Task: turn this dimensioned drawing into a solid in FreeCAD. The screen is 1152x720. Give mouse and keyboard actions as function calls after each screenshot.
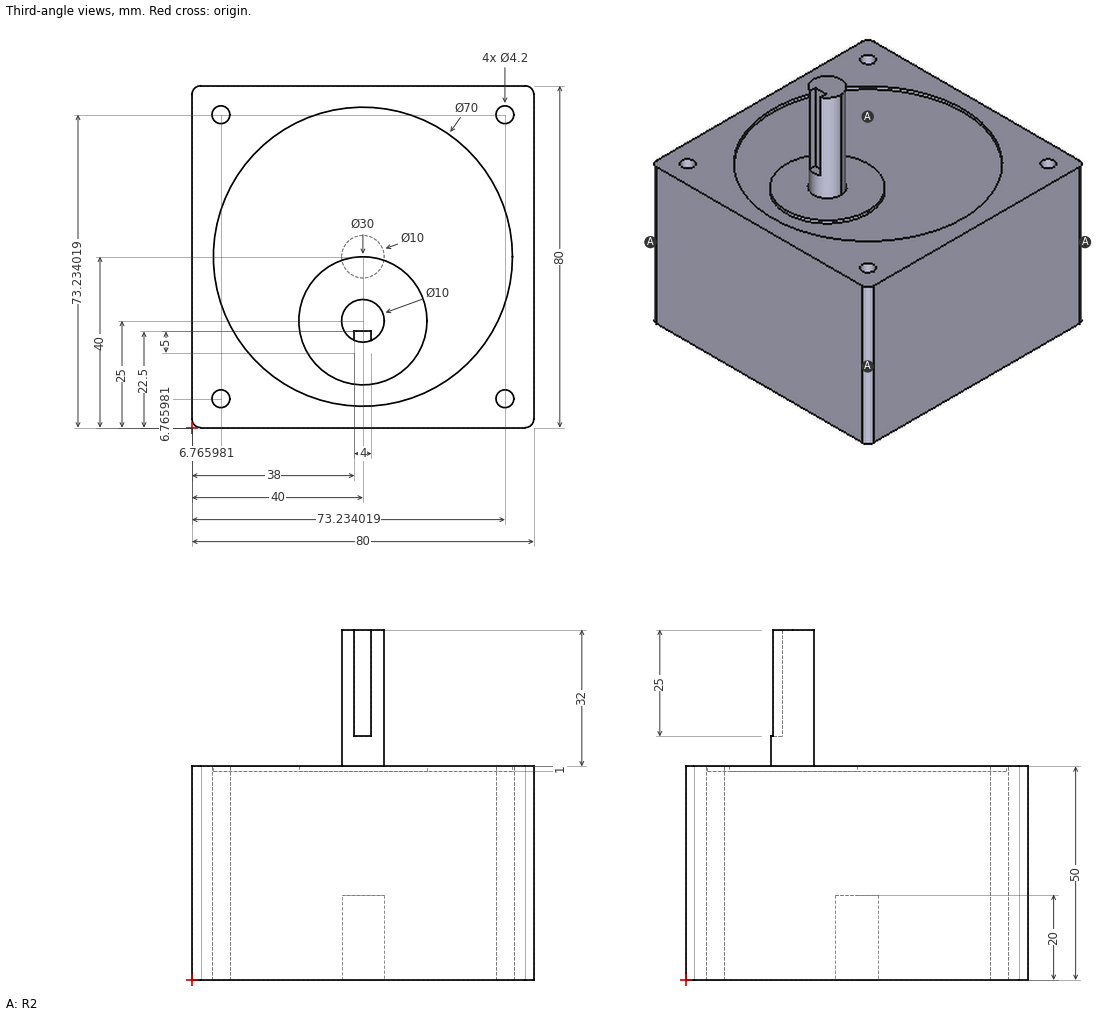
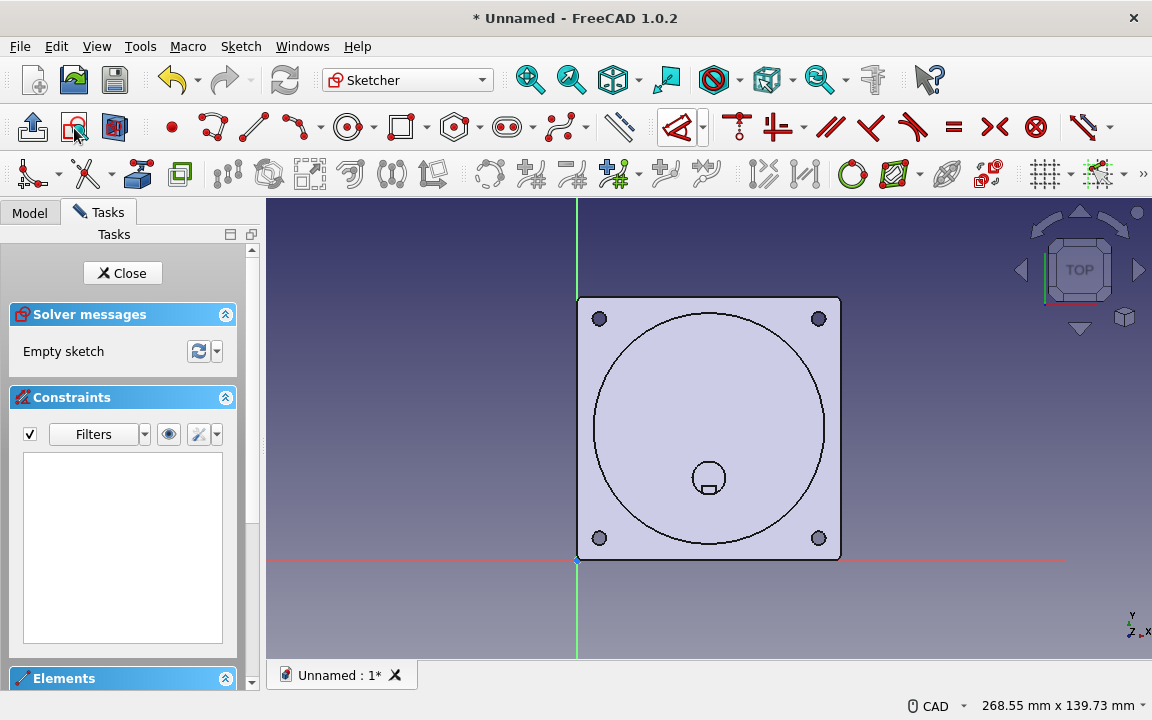
scroll(690, 548, up, 4)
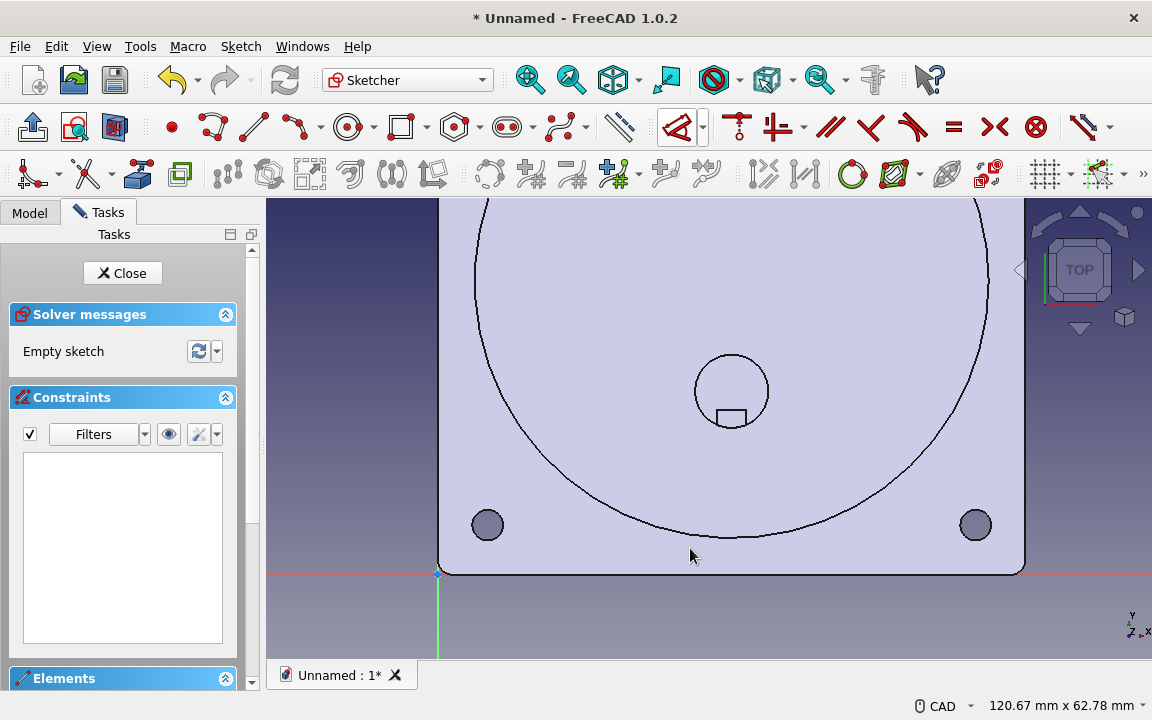
click(348, 128)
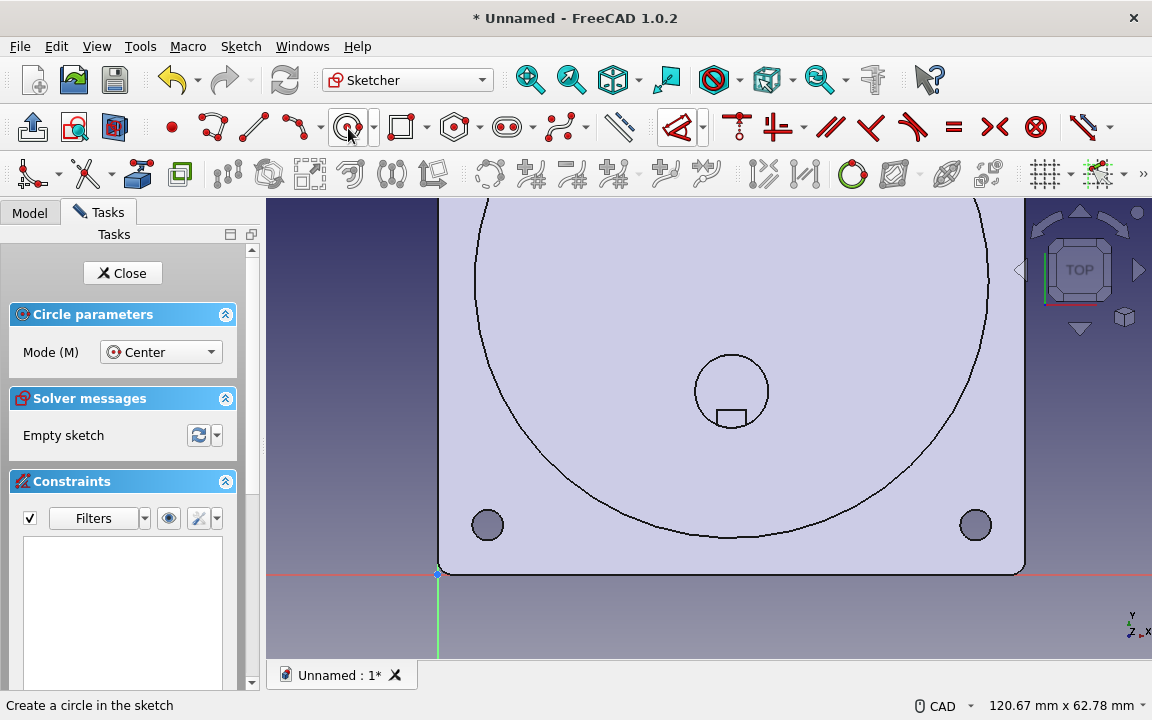
click(732, 391)
click(810, 313)
key(Escape)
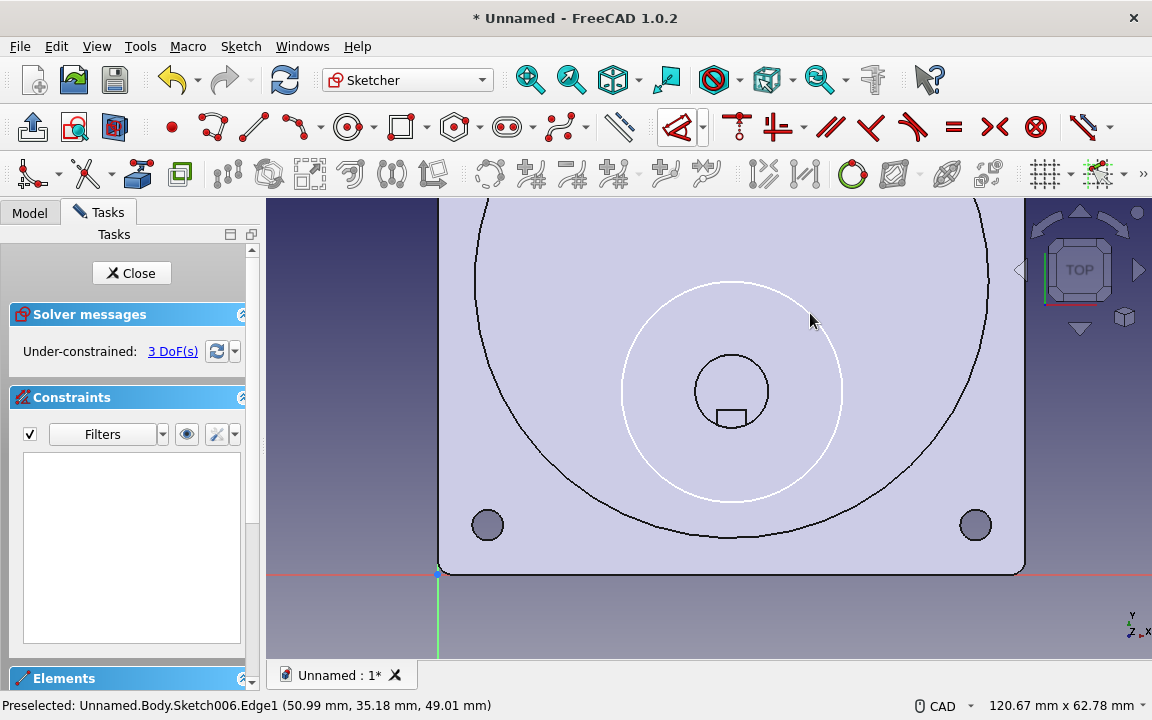
click(810, 314)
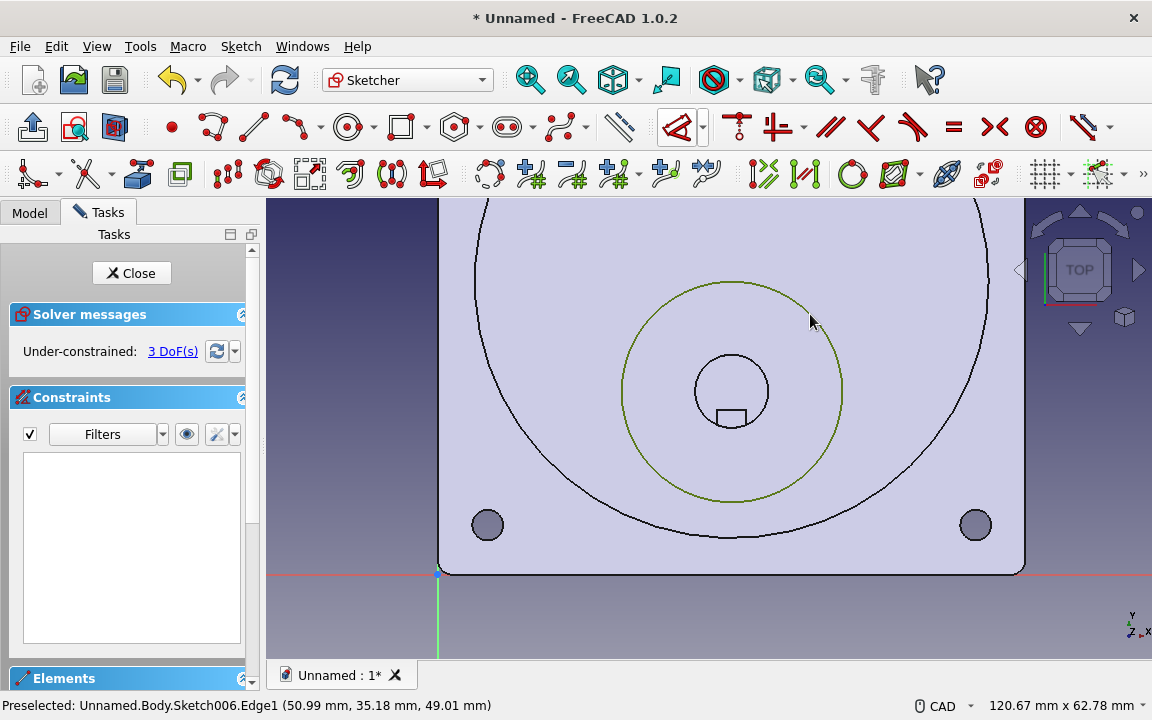
click(702, 128)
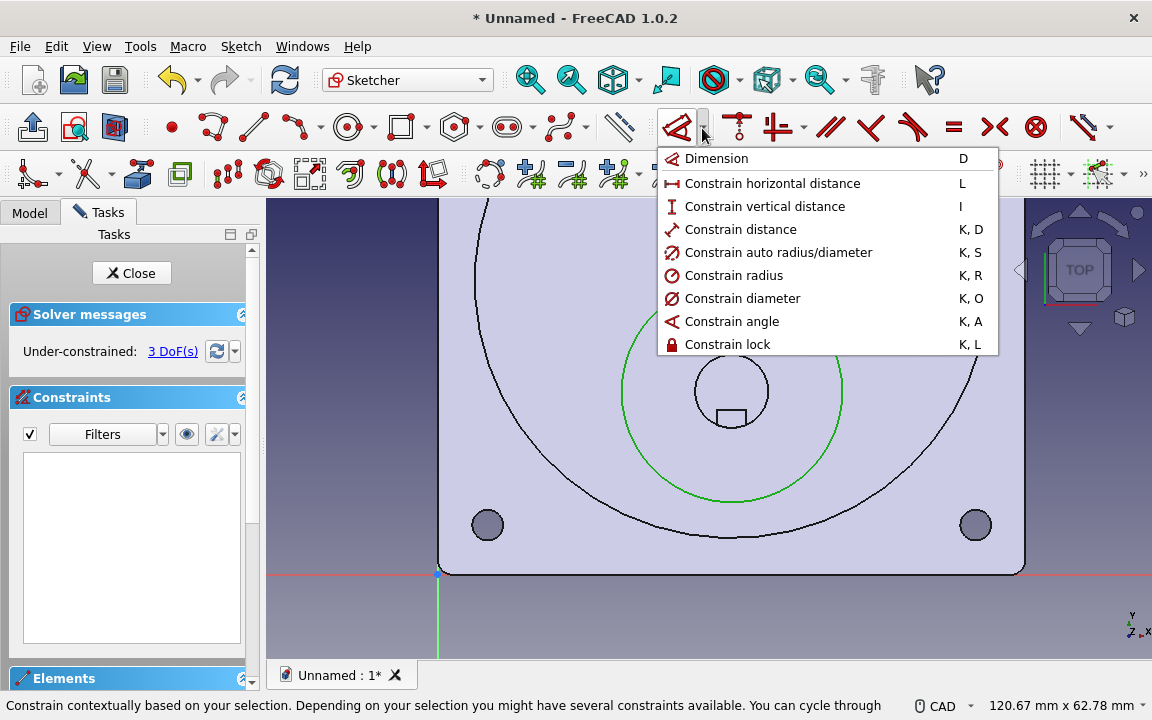
click(828, 298)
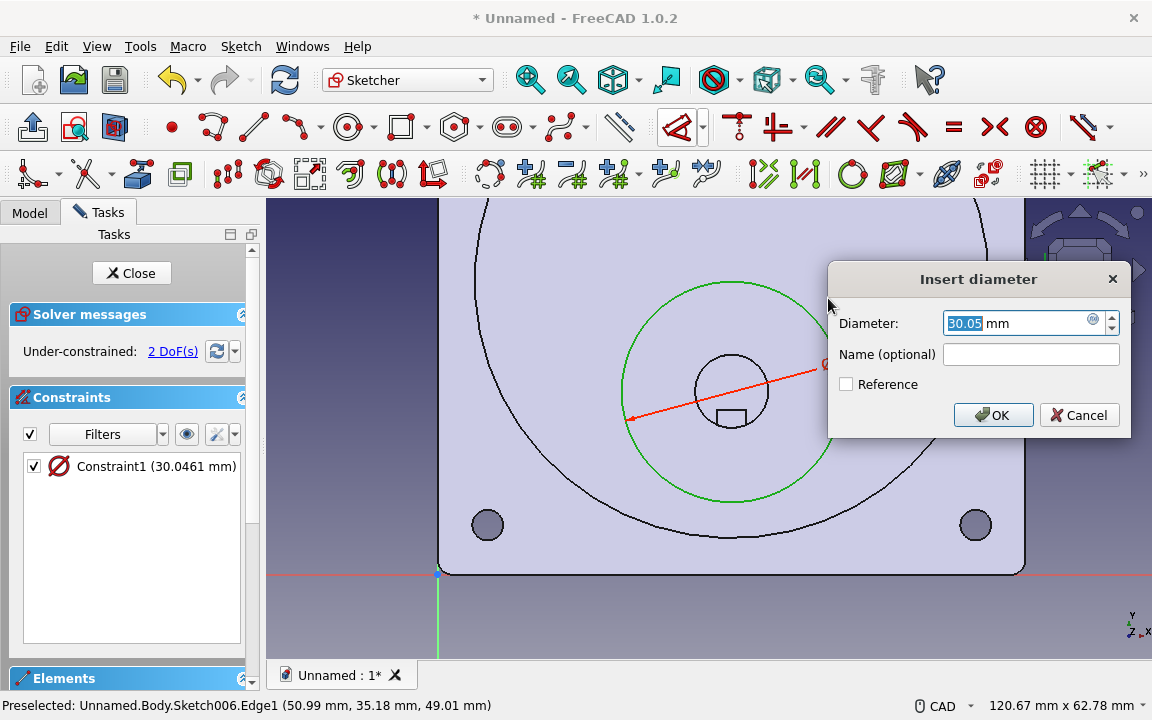
text(30)
key(Return)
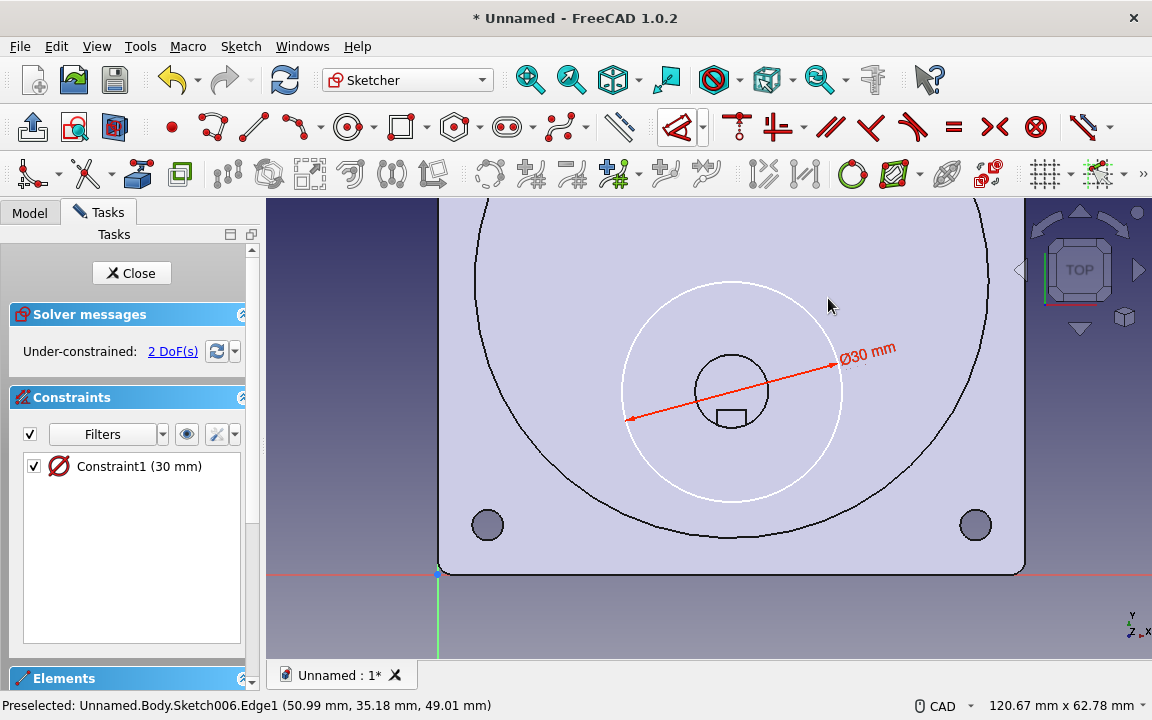
click(732, 392)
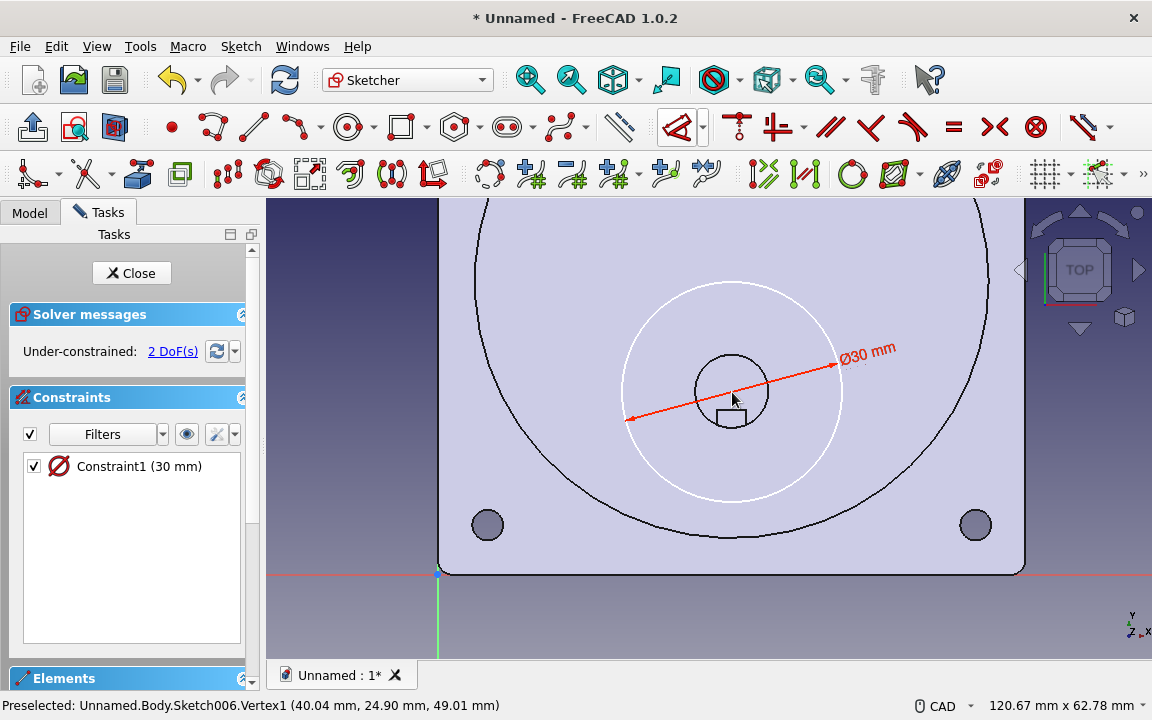
key(l)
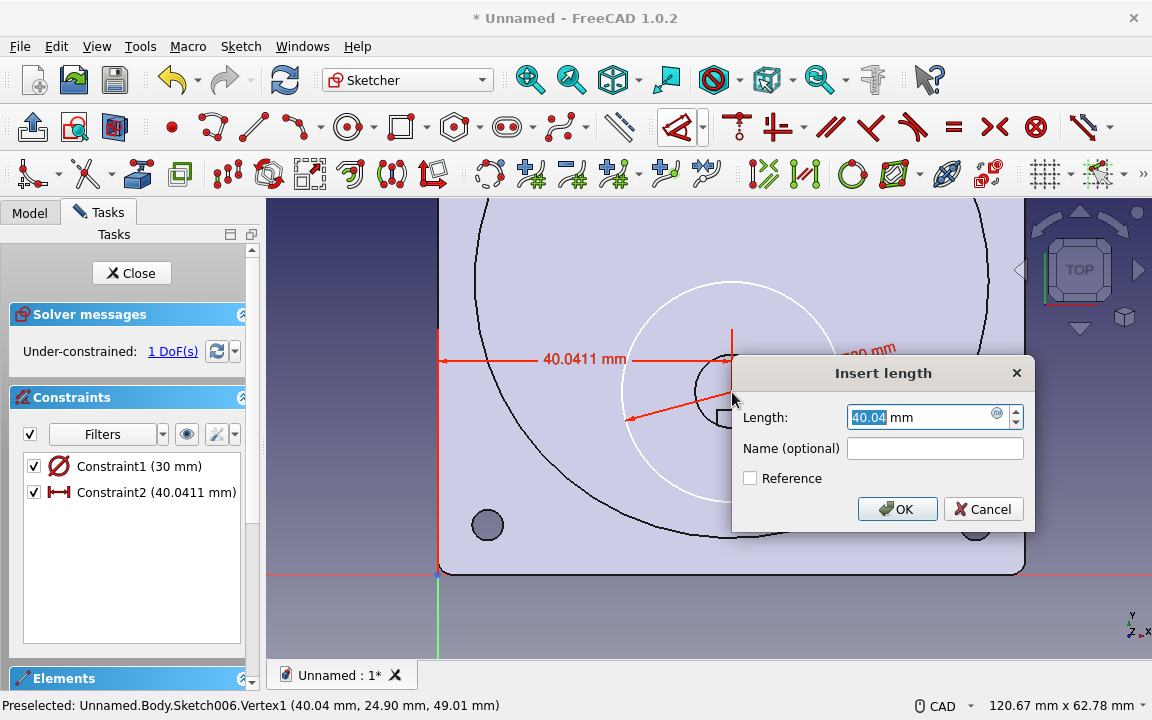
text(40)
key(Return)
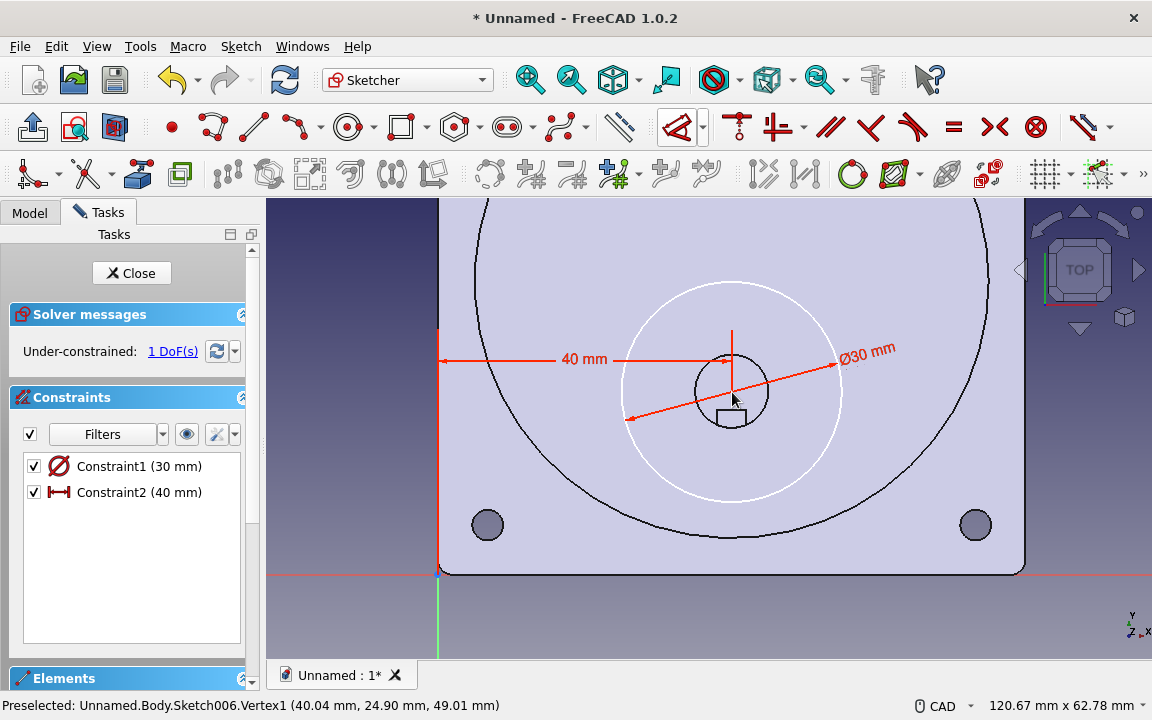
click(732, 392)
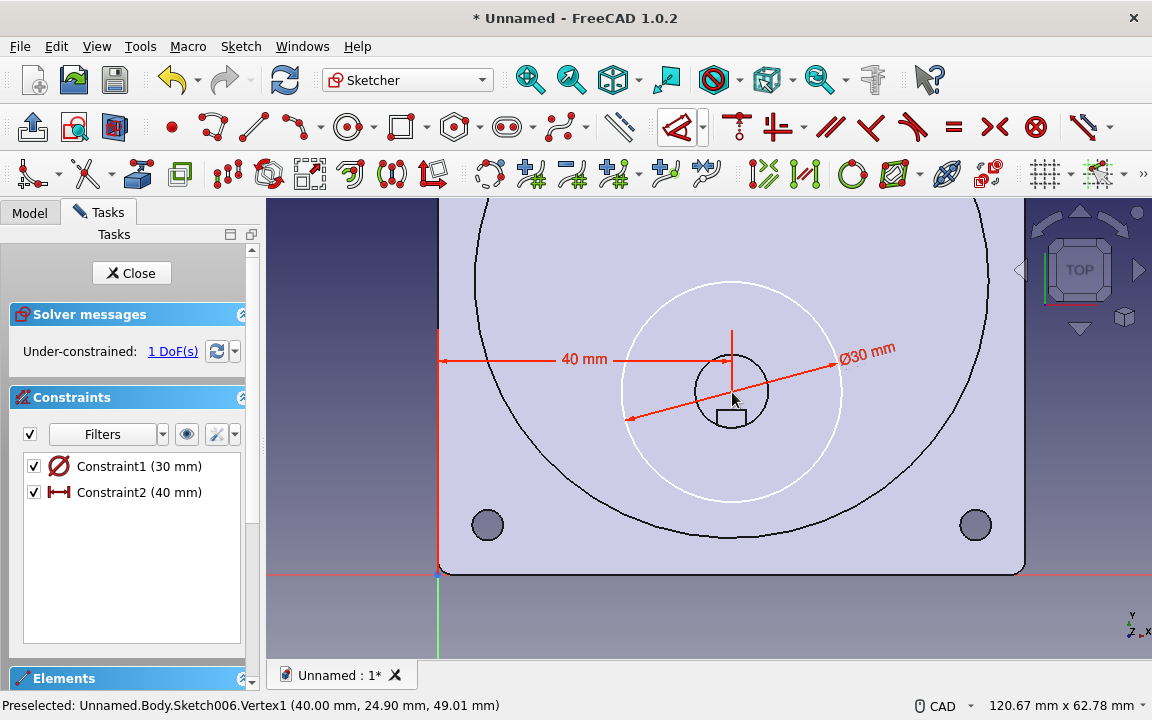
click(702, 128)